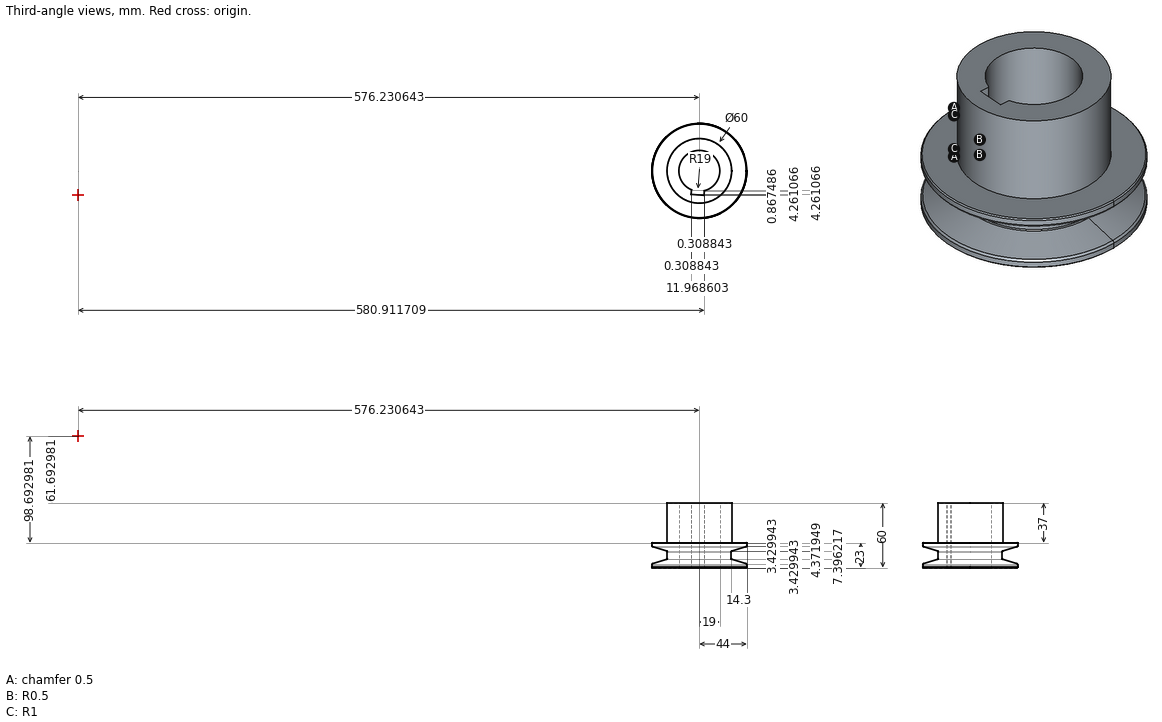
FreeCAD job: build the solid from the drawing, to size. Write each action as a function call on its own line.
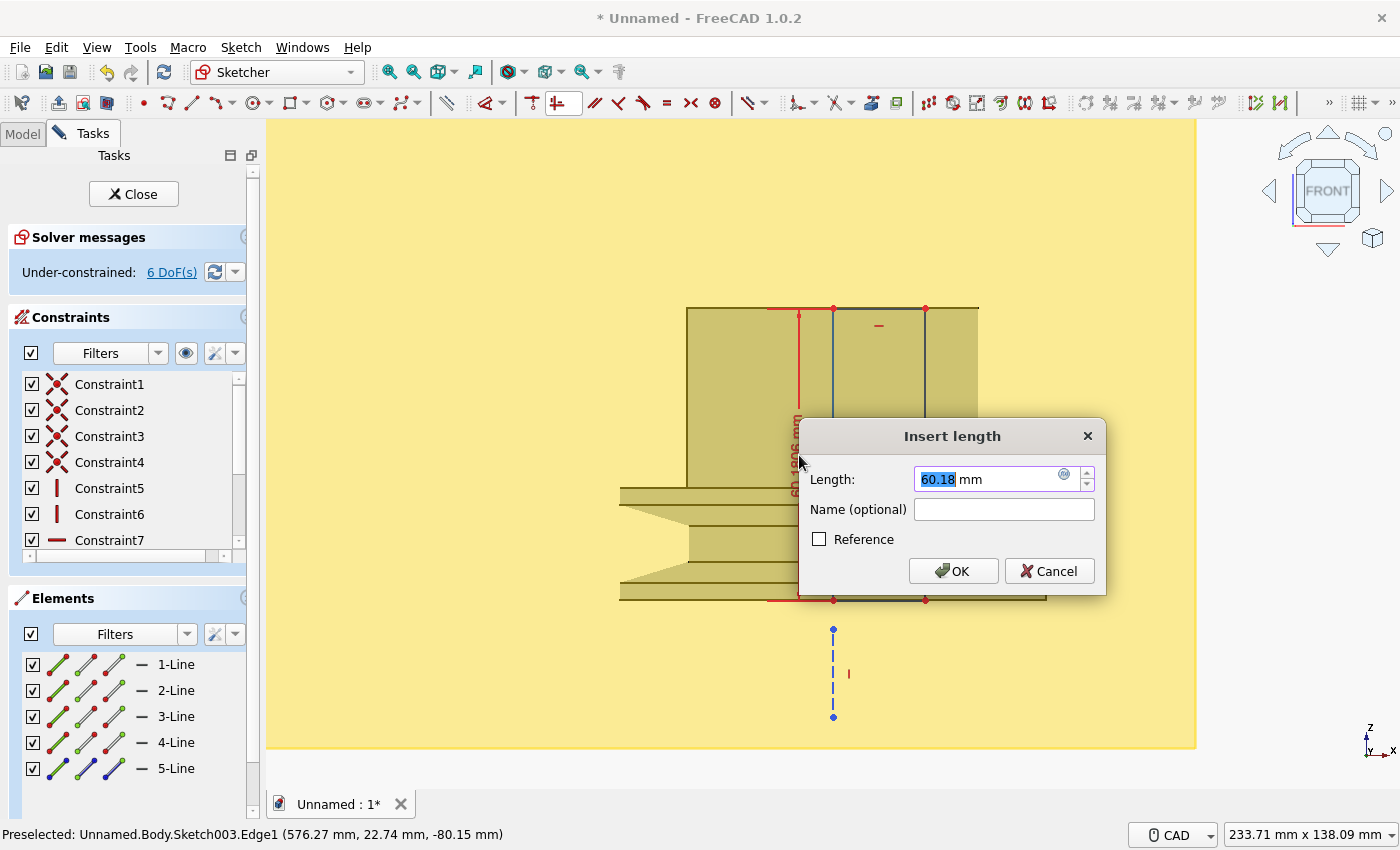
text(60)
key(Return)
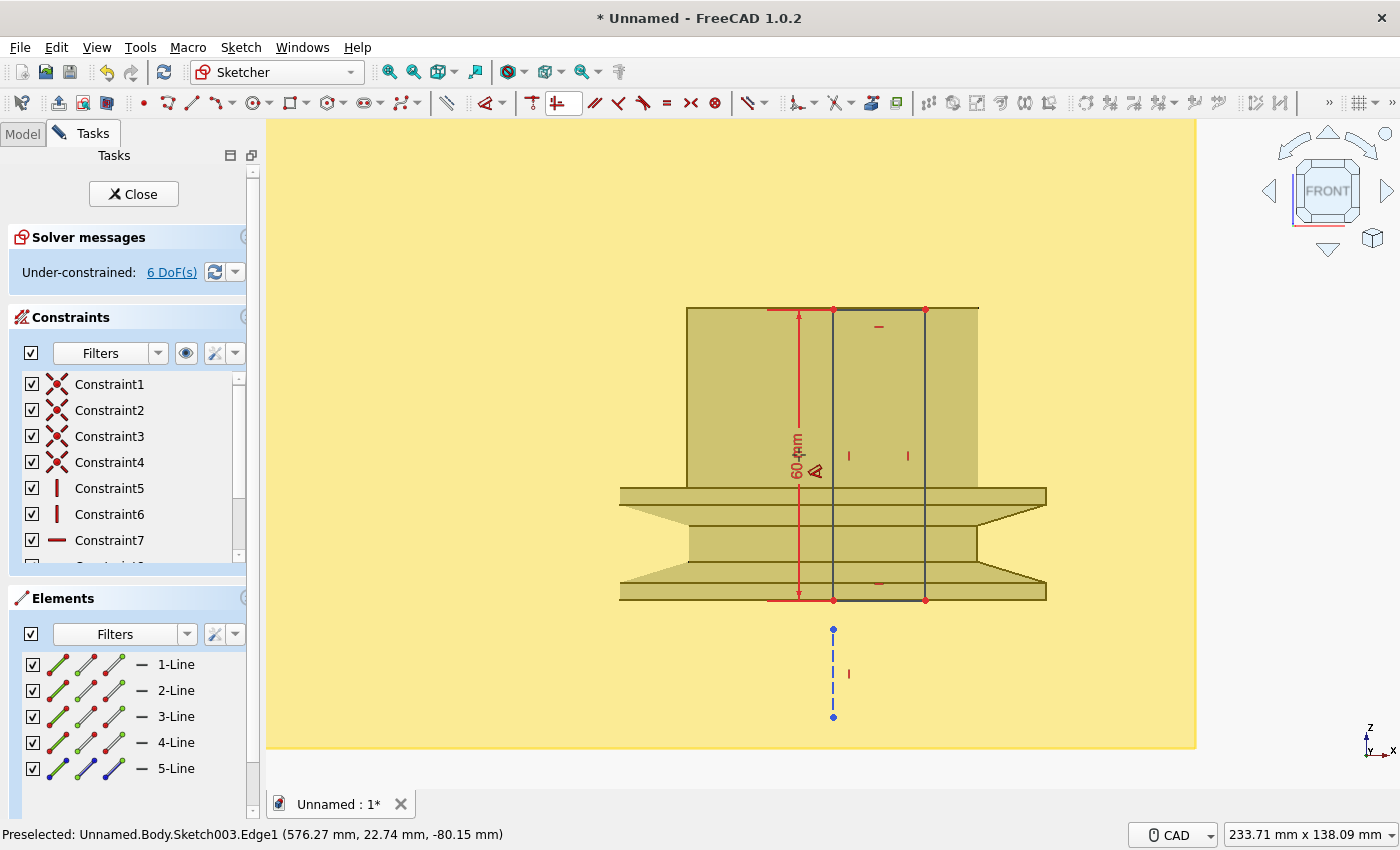
click(861, 601)
click(879, 635)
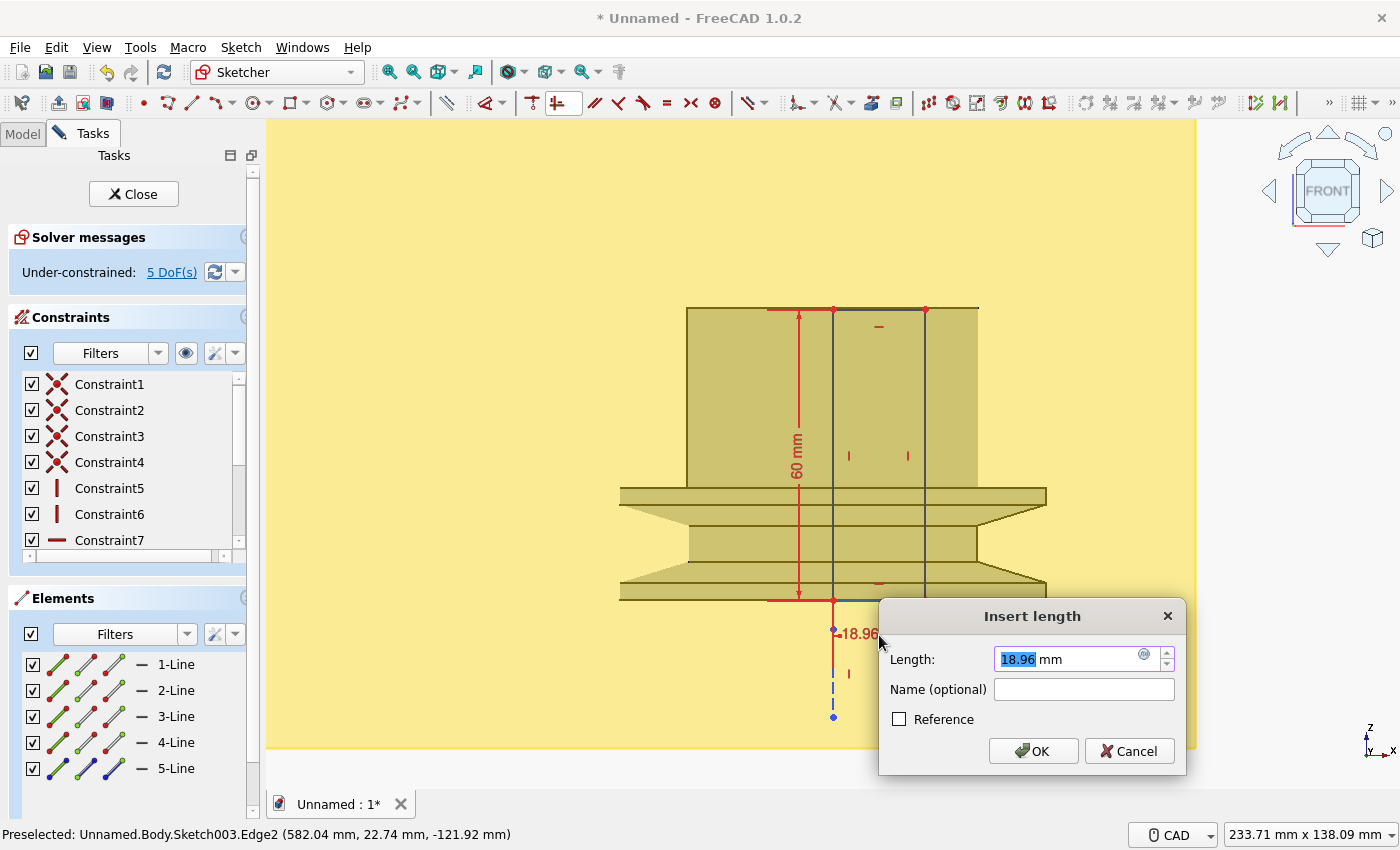
text(19)
key(Return)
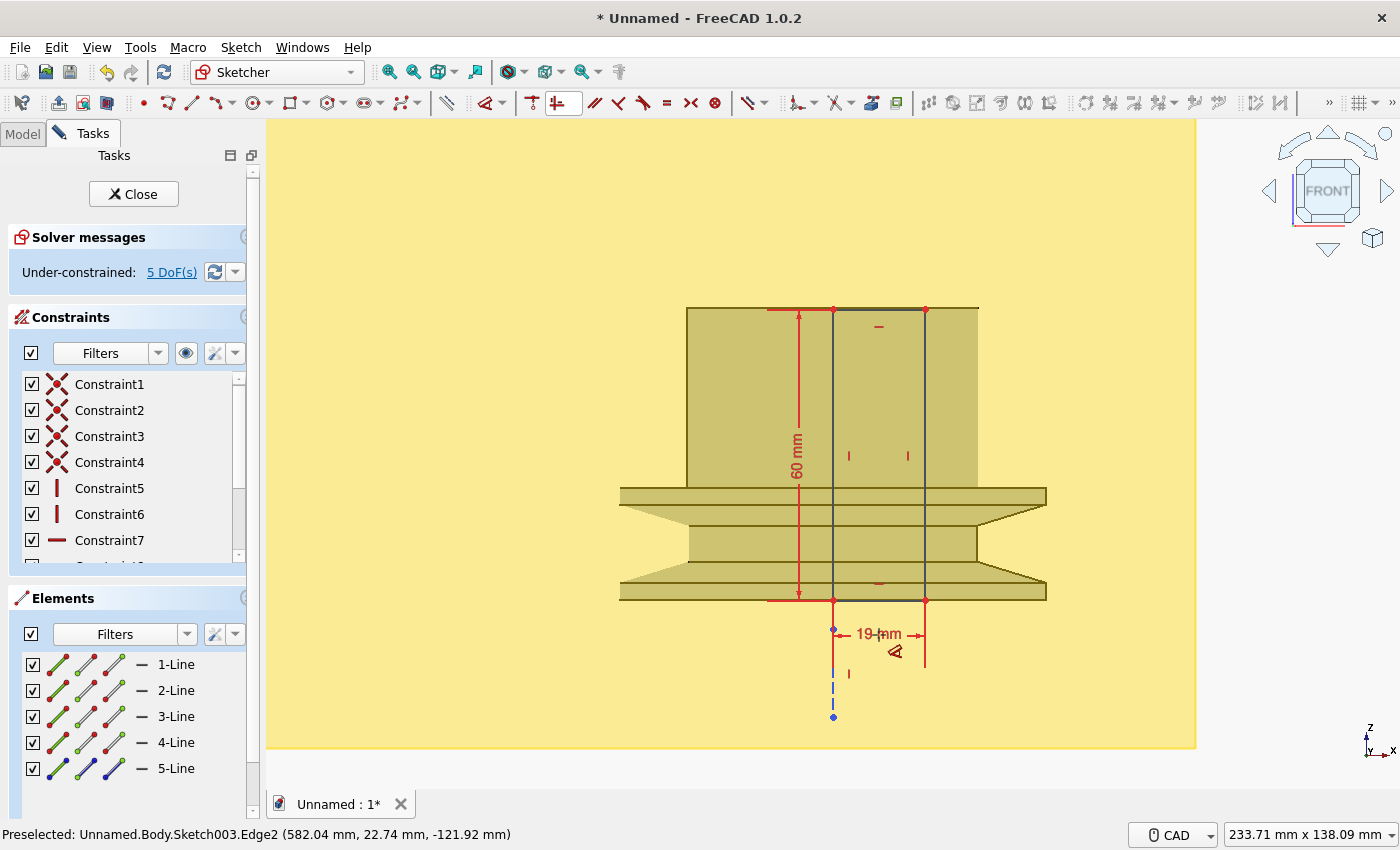
click(833, 310)
click(867, 228)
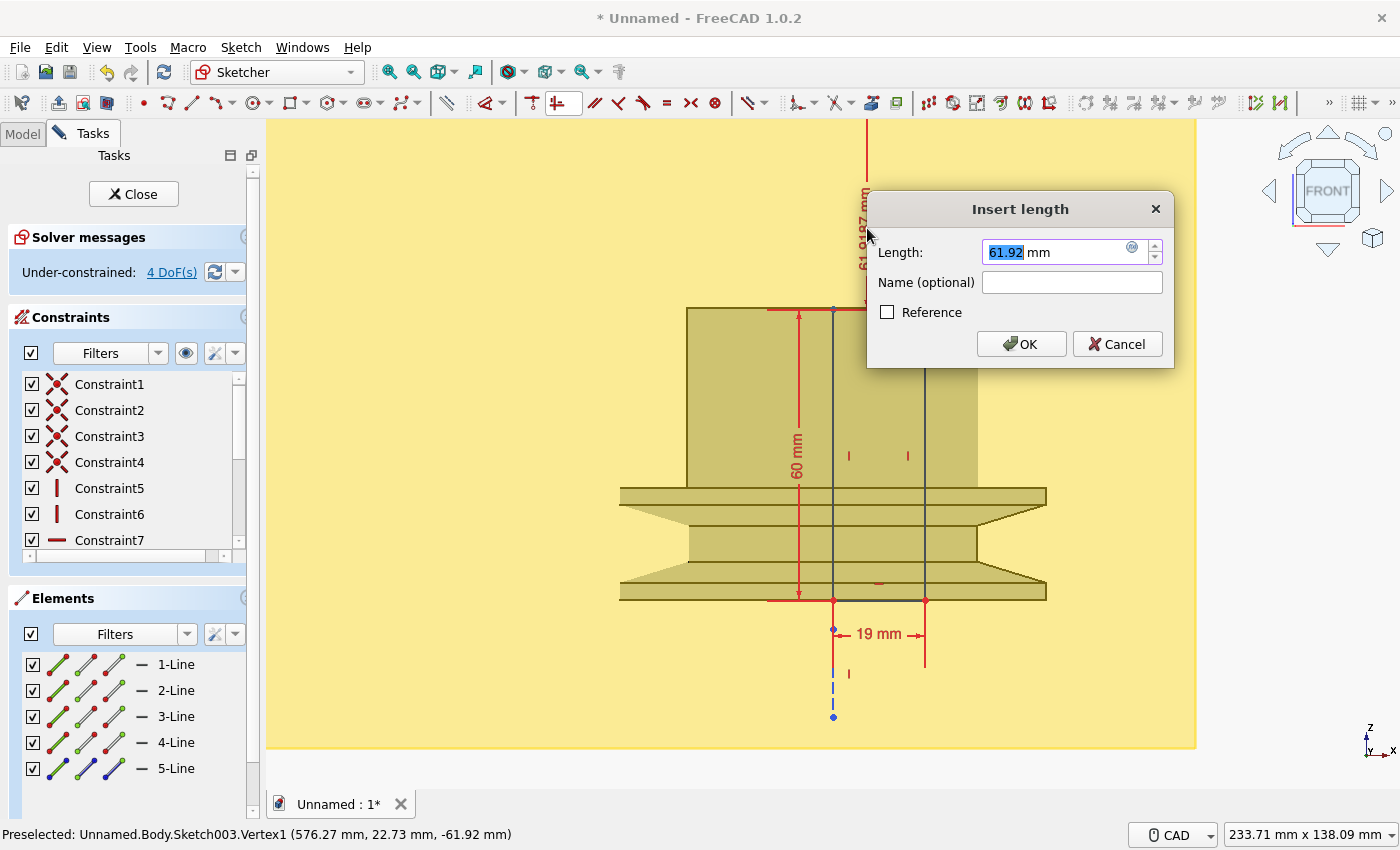
text(61.692981)
key(Return)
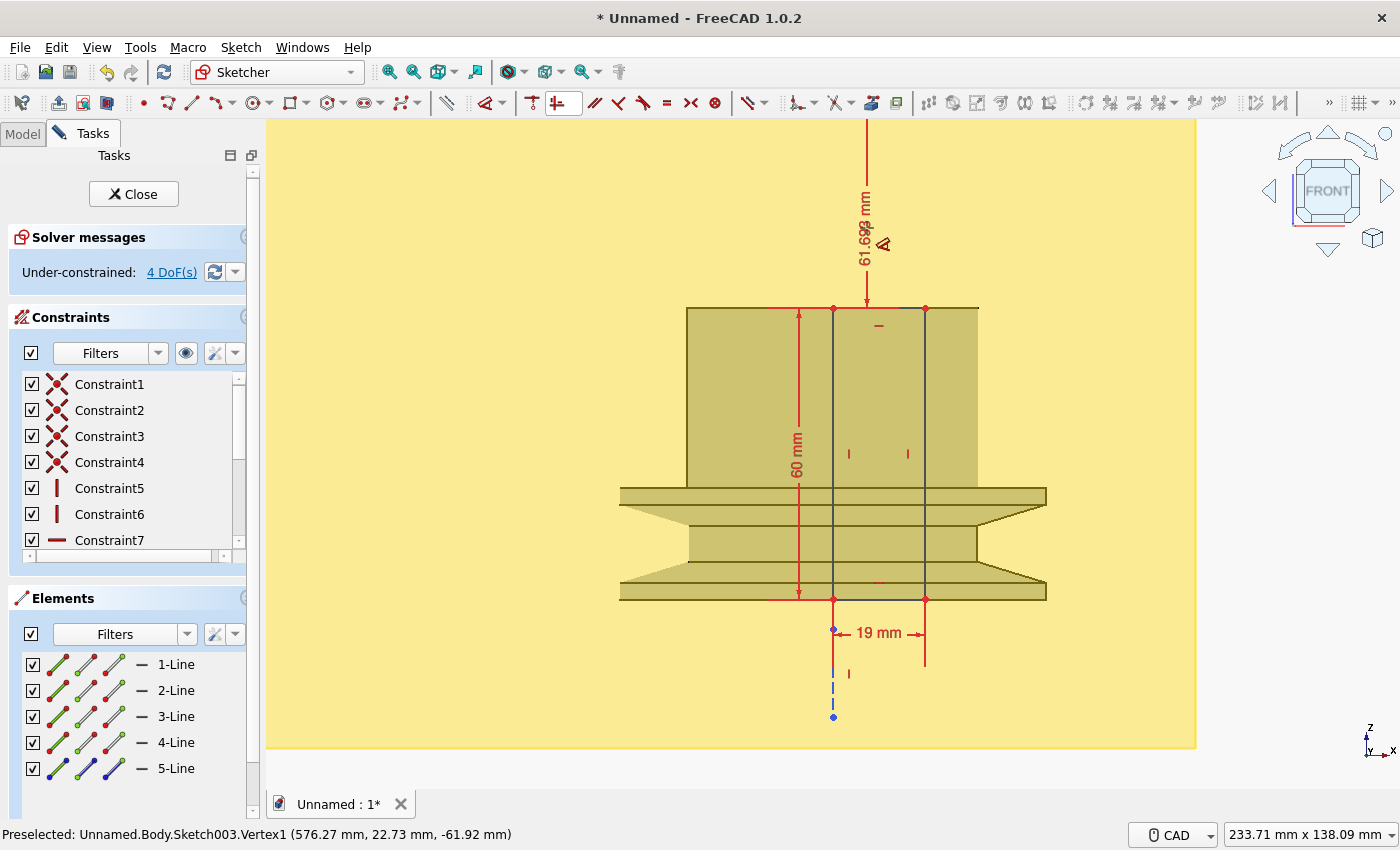
click(833, 308)
click(563, 342)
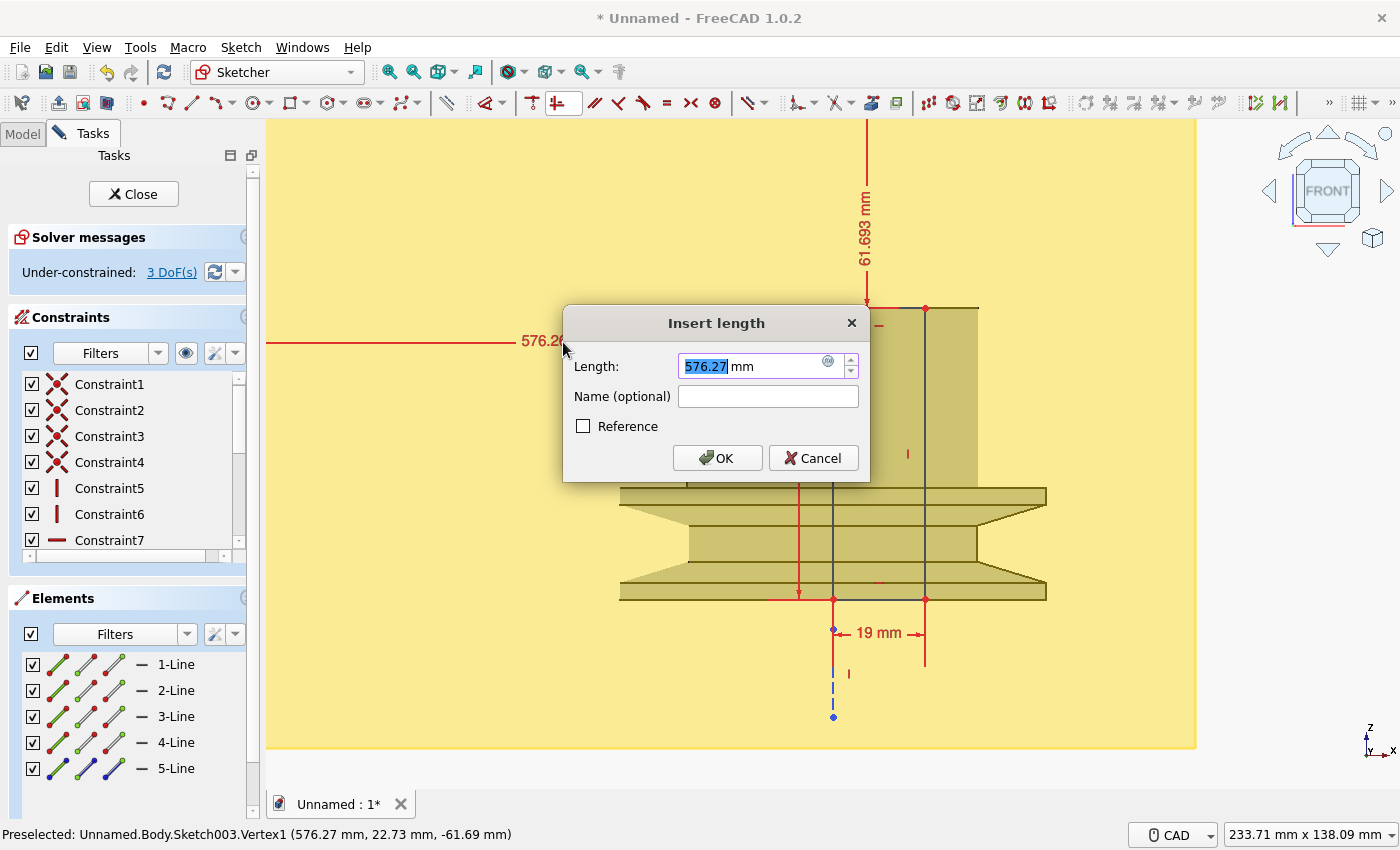
text(576.230643)
key(Return)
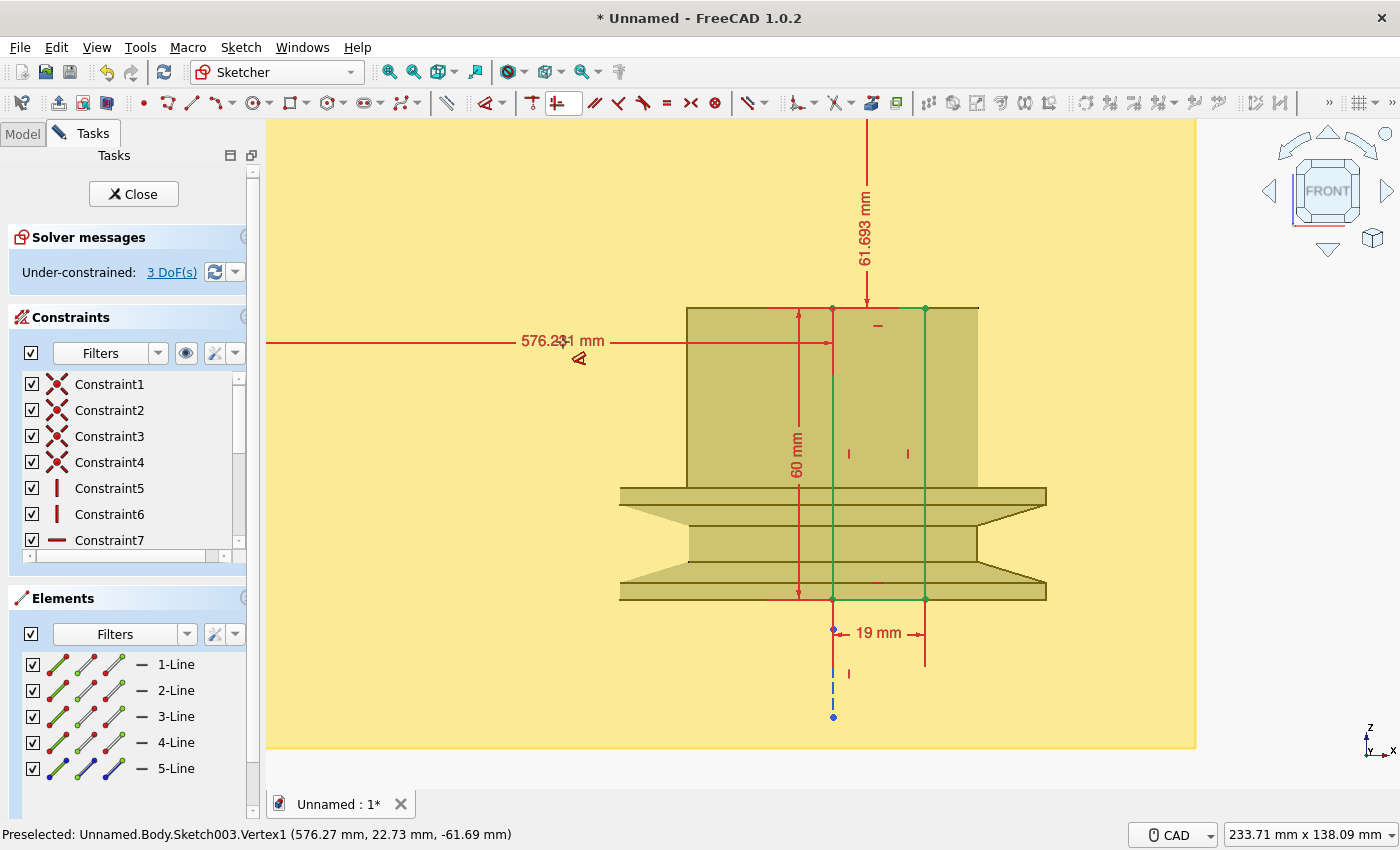
click(833, 630)
click(563, 664)